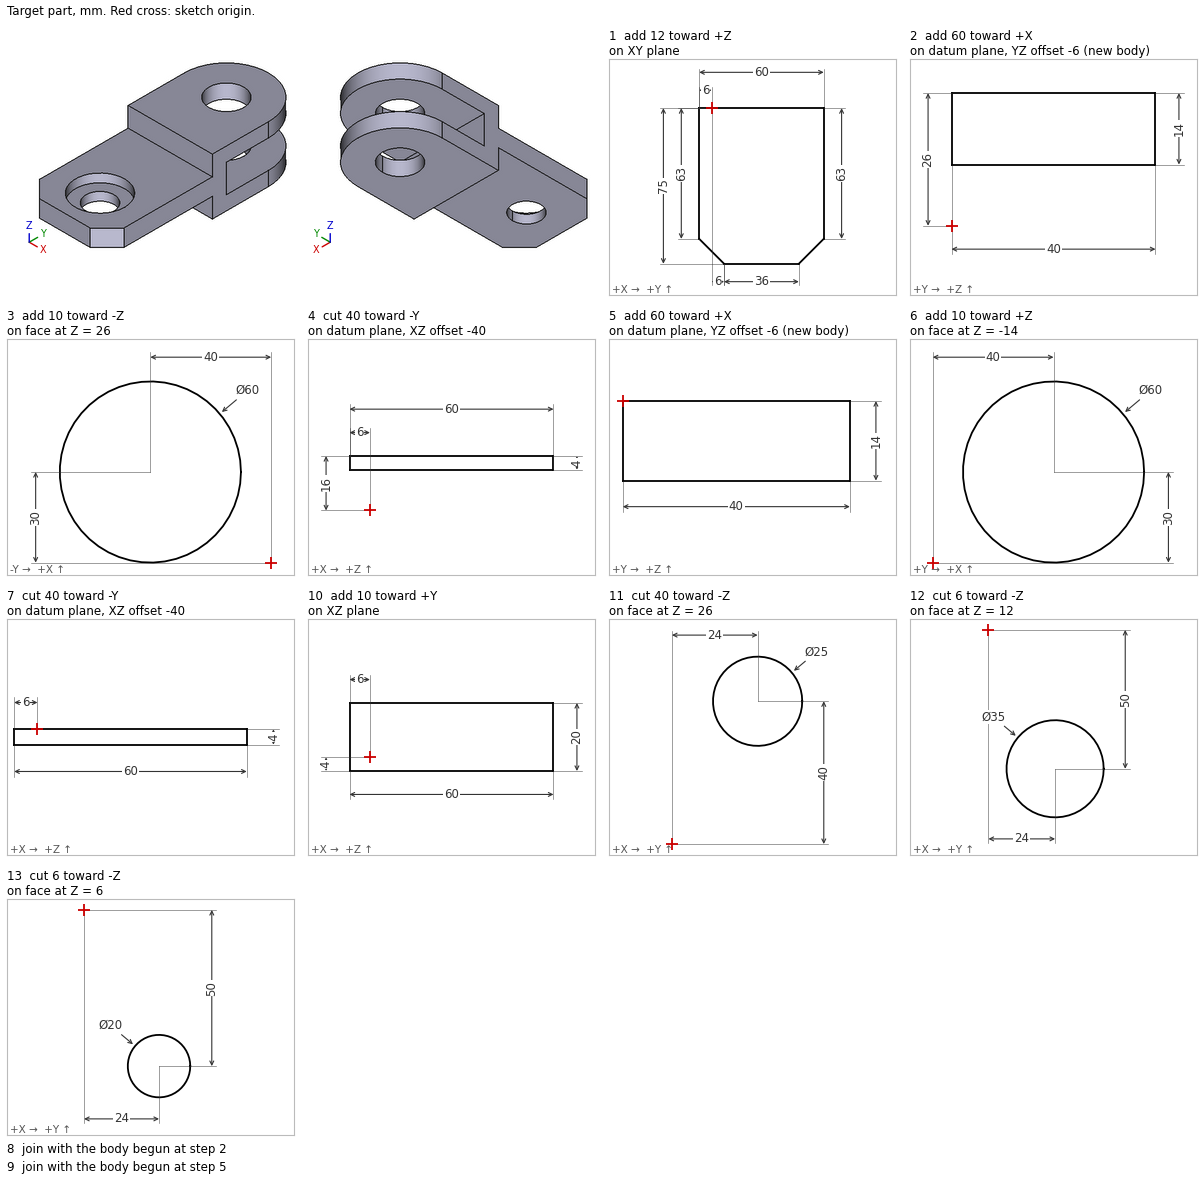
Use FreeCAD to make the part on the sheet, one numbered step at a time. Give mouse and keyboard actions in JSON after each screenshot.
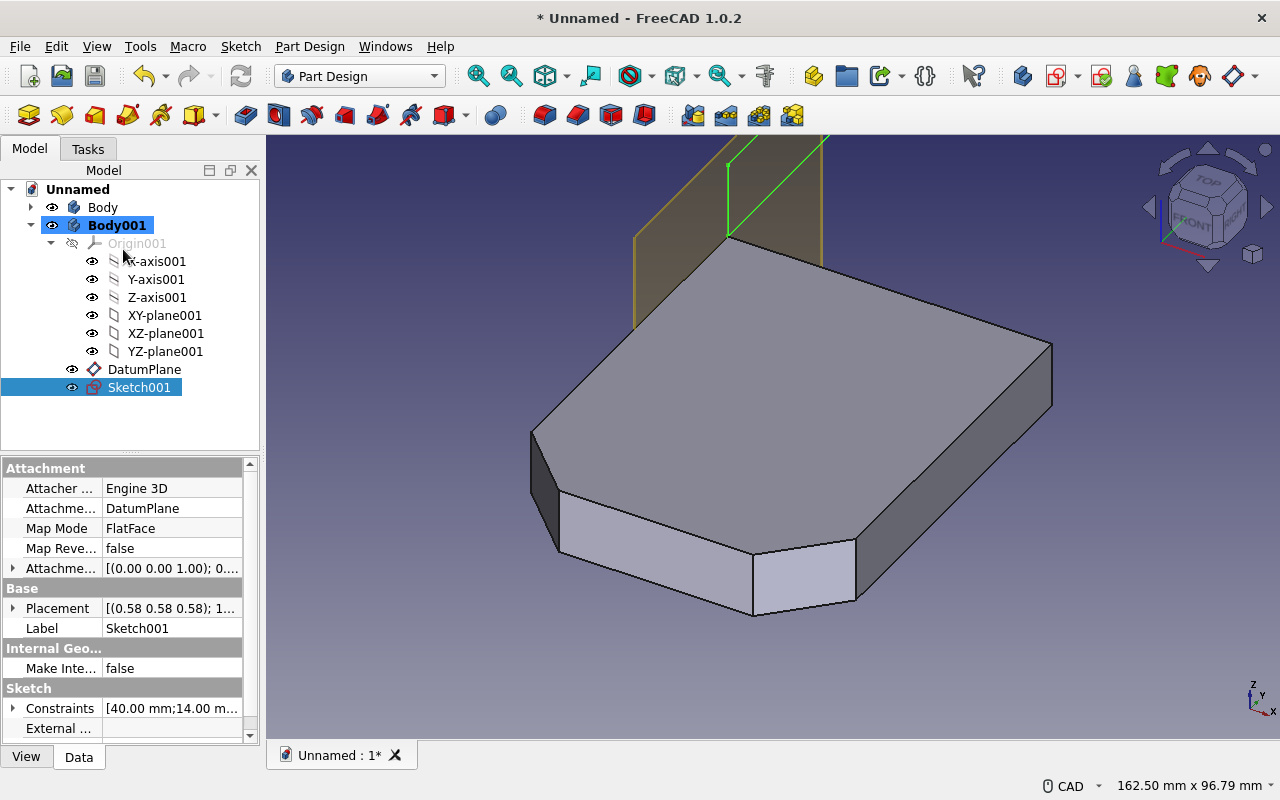
{"action": "left_click", "coordinate": [29, 116]}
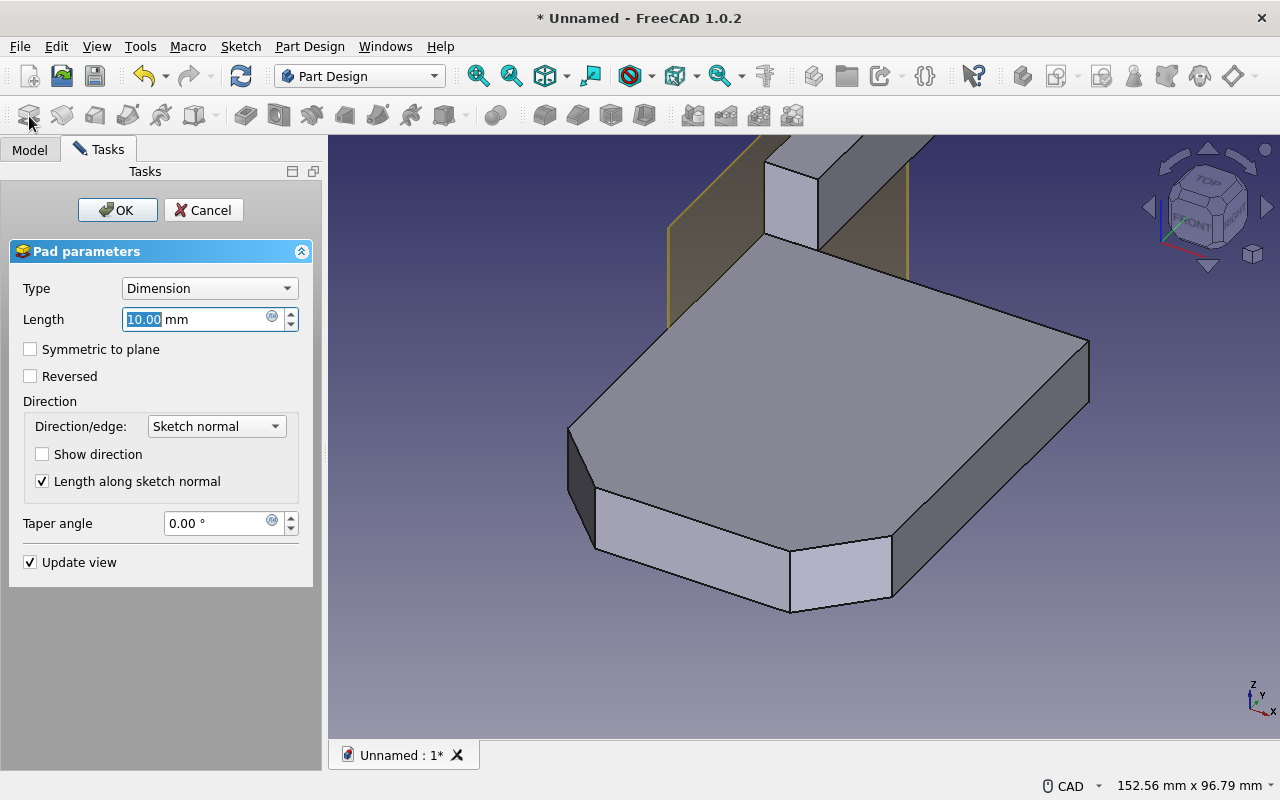
{"action": "type", "text": "60"}
{"action": "key", "text": "Tab"}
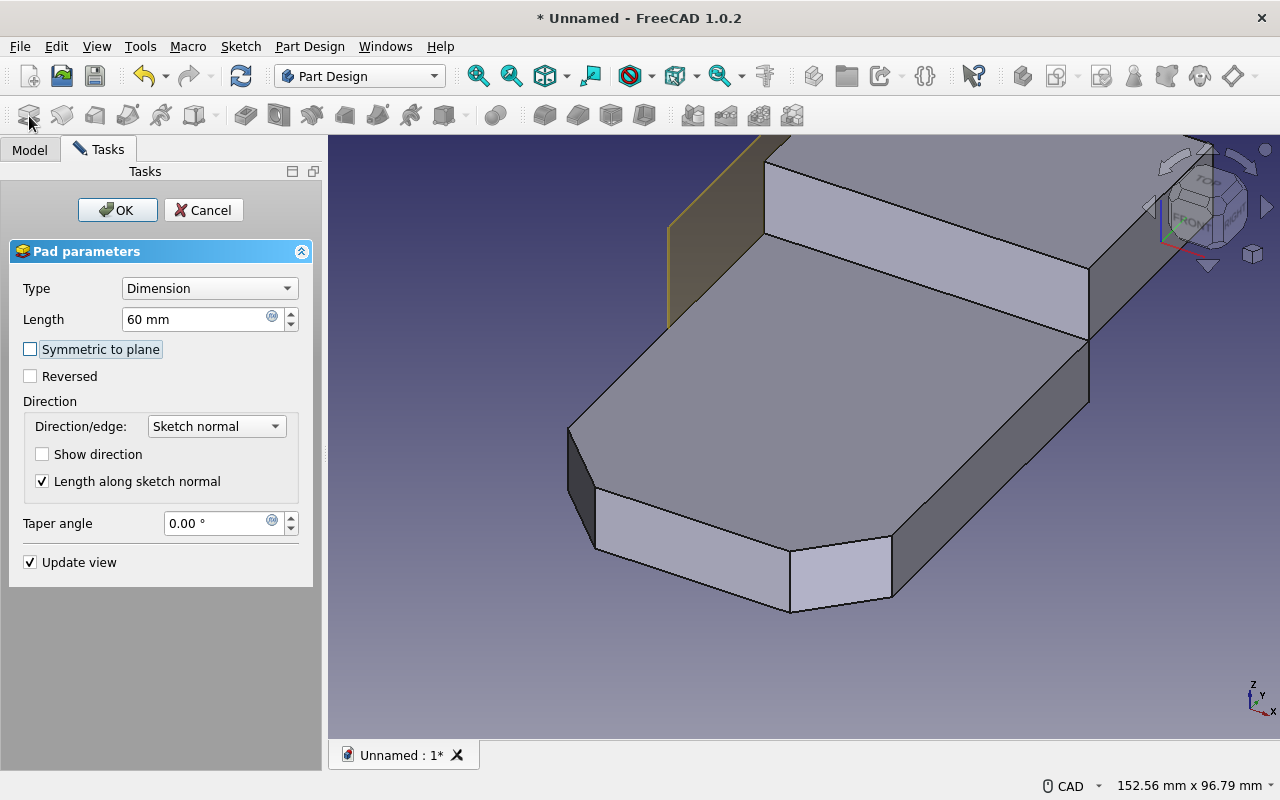
{"action": "left_click", "coordinate": [118, 210]}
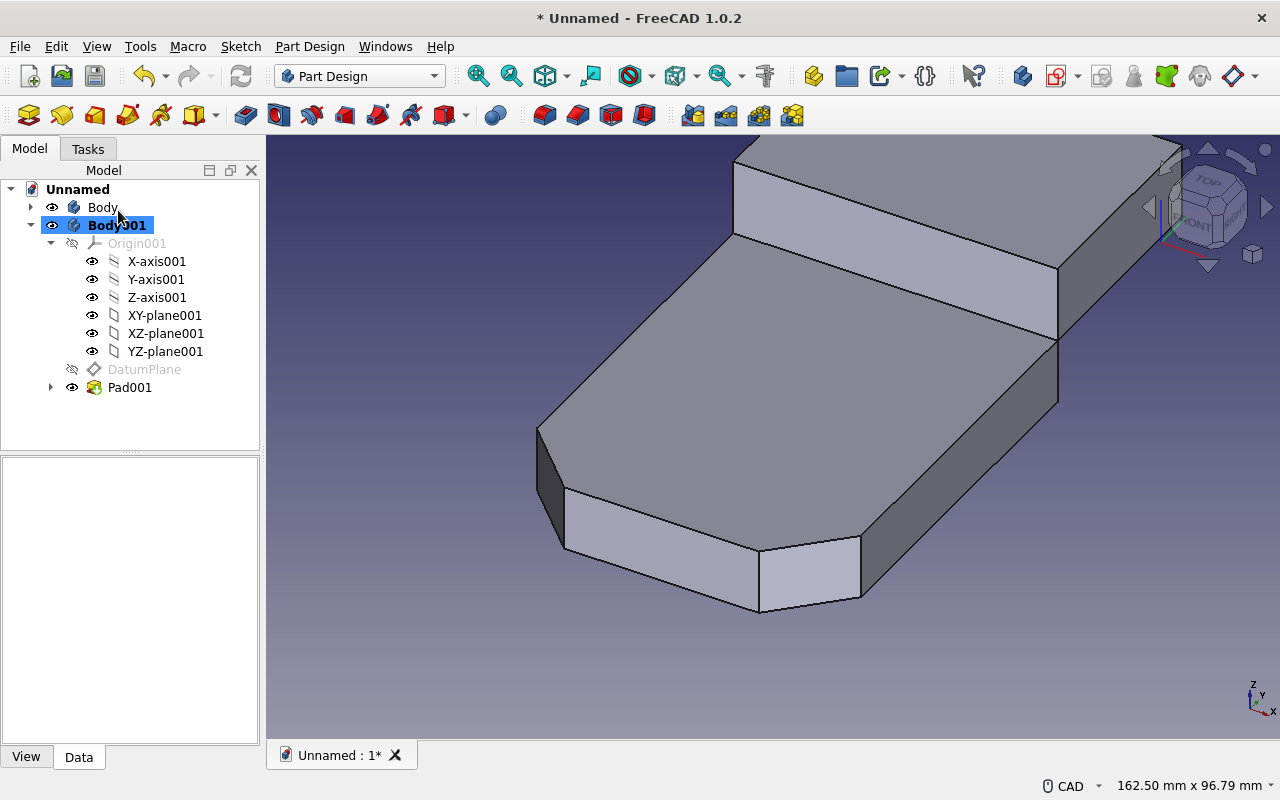
{"action": "left_click", "coordinate": [479, 76]}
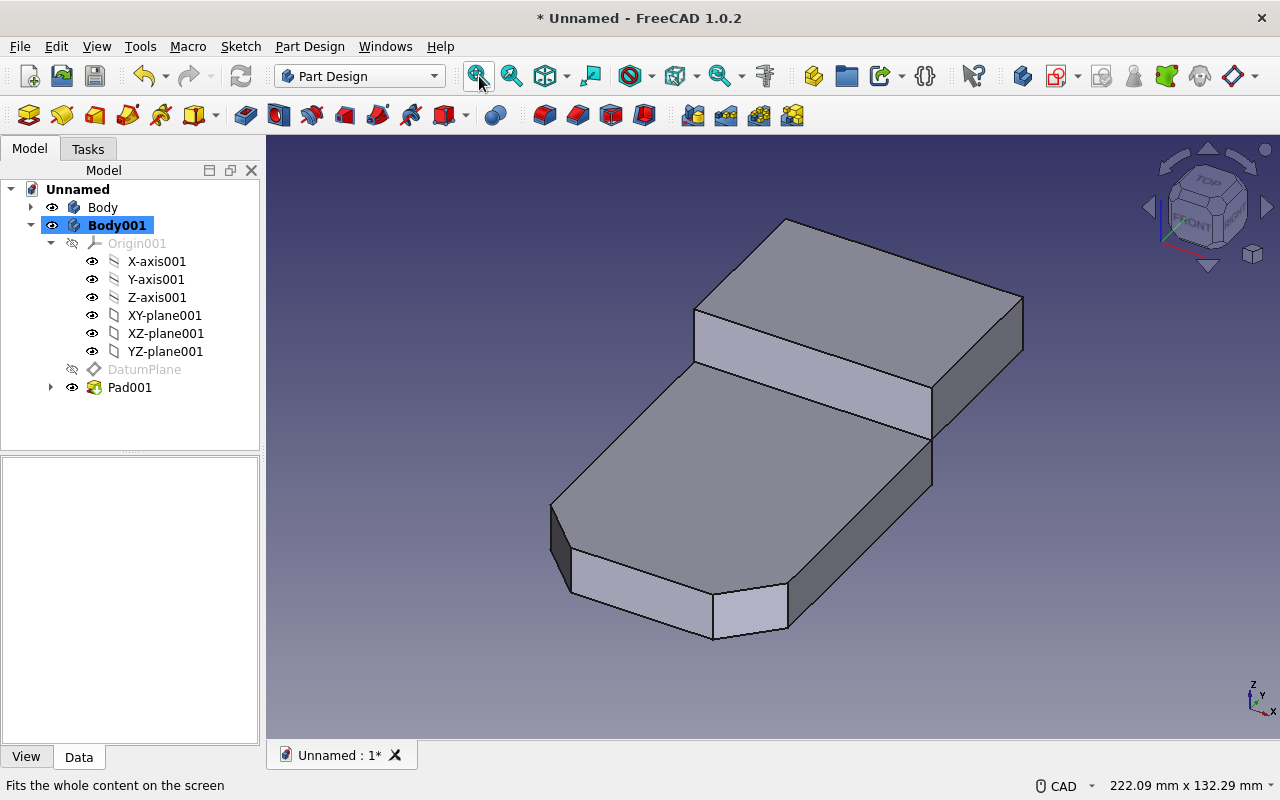
{"action": "left_click", "coordinate": [892, 314]}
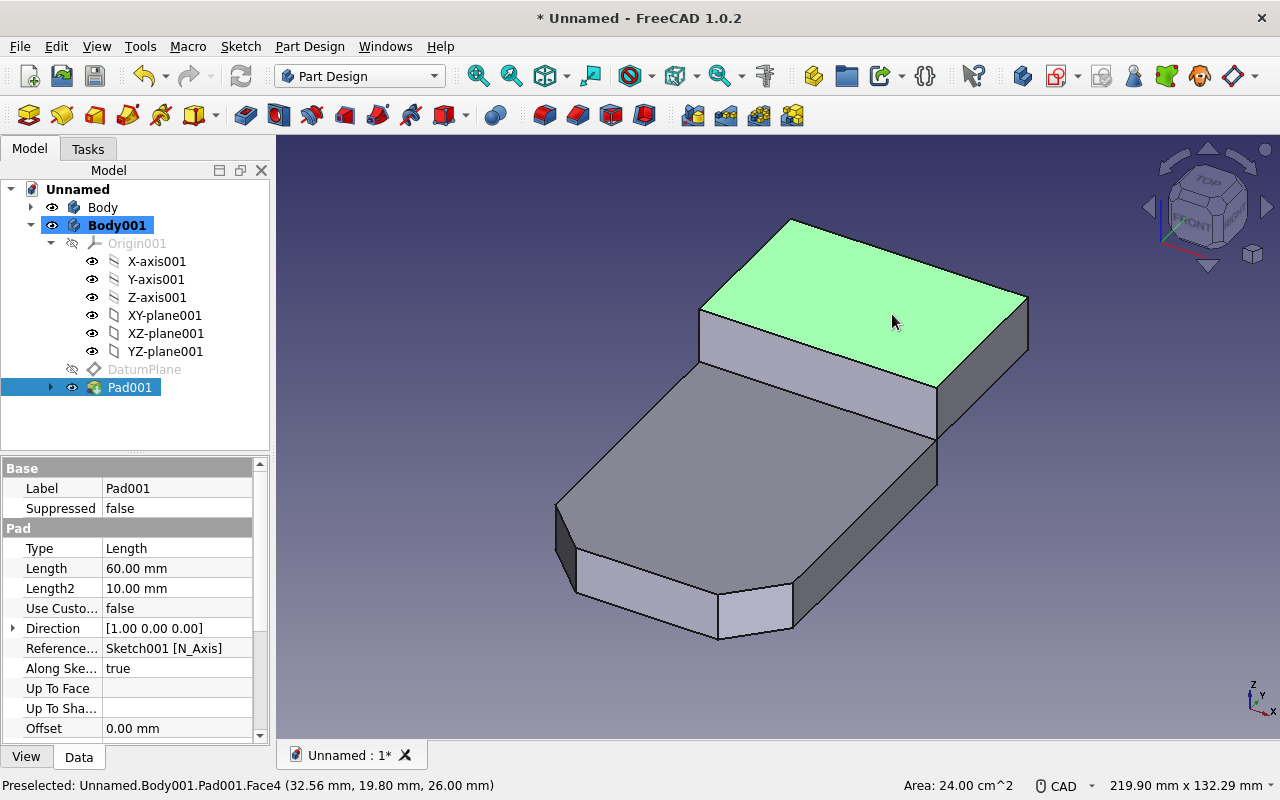
{"action": "left_click", "coordinate": [1056, 76]}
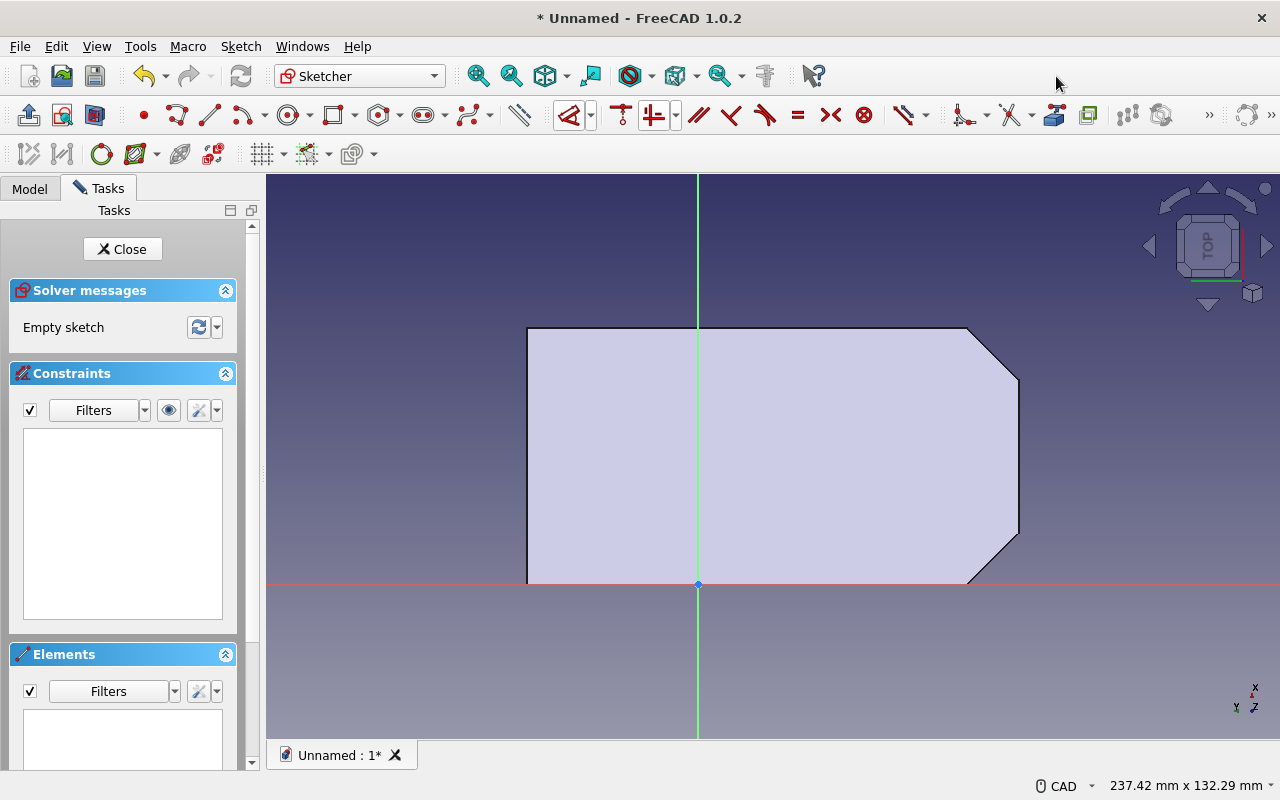
{"action": "scroll", "coordinate": [294, 457], "scroll_direction": "up", "scroll_amount": 2}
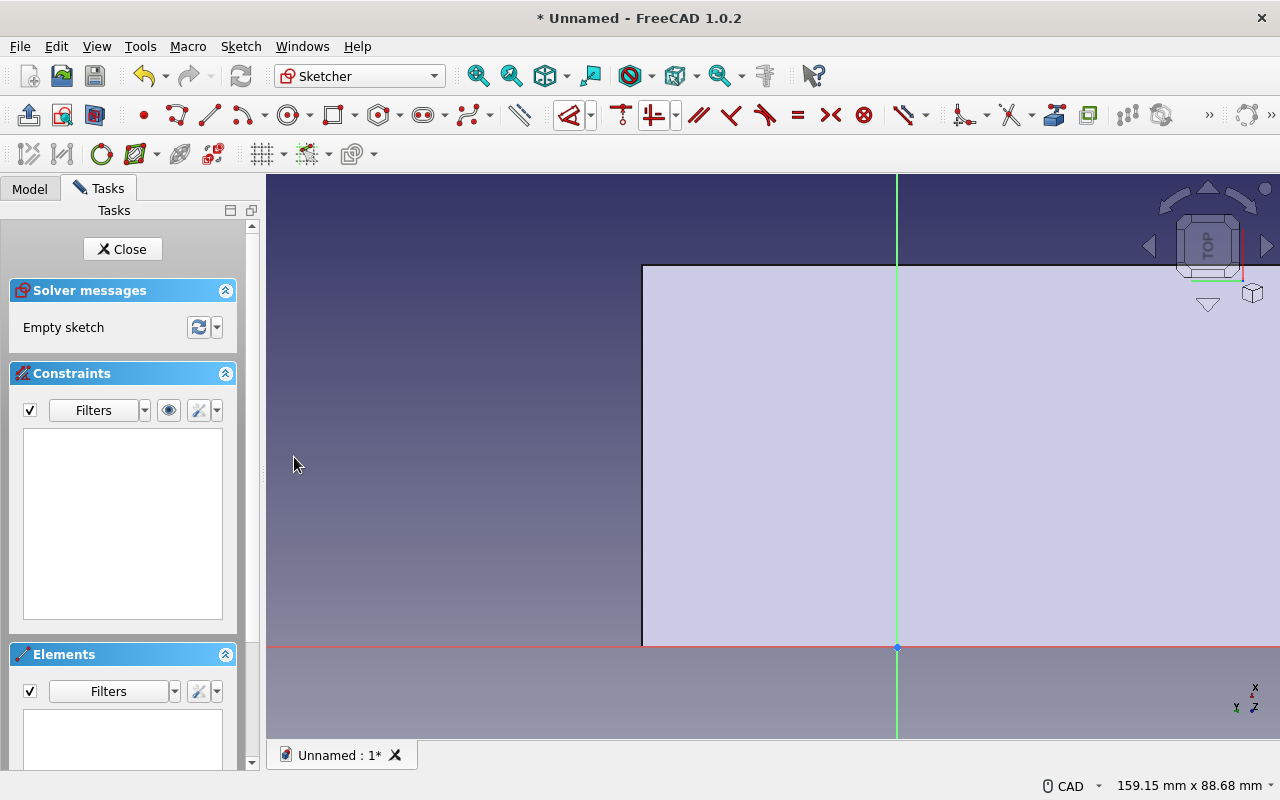
{"action": "left_click", "coordinate": [288, 116]}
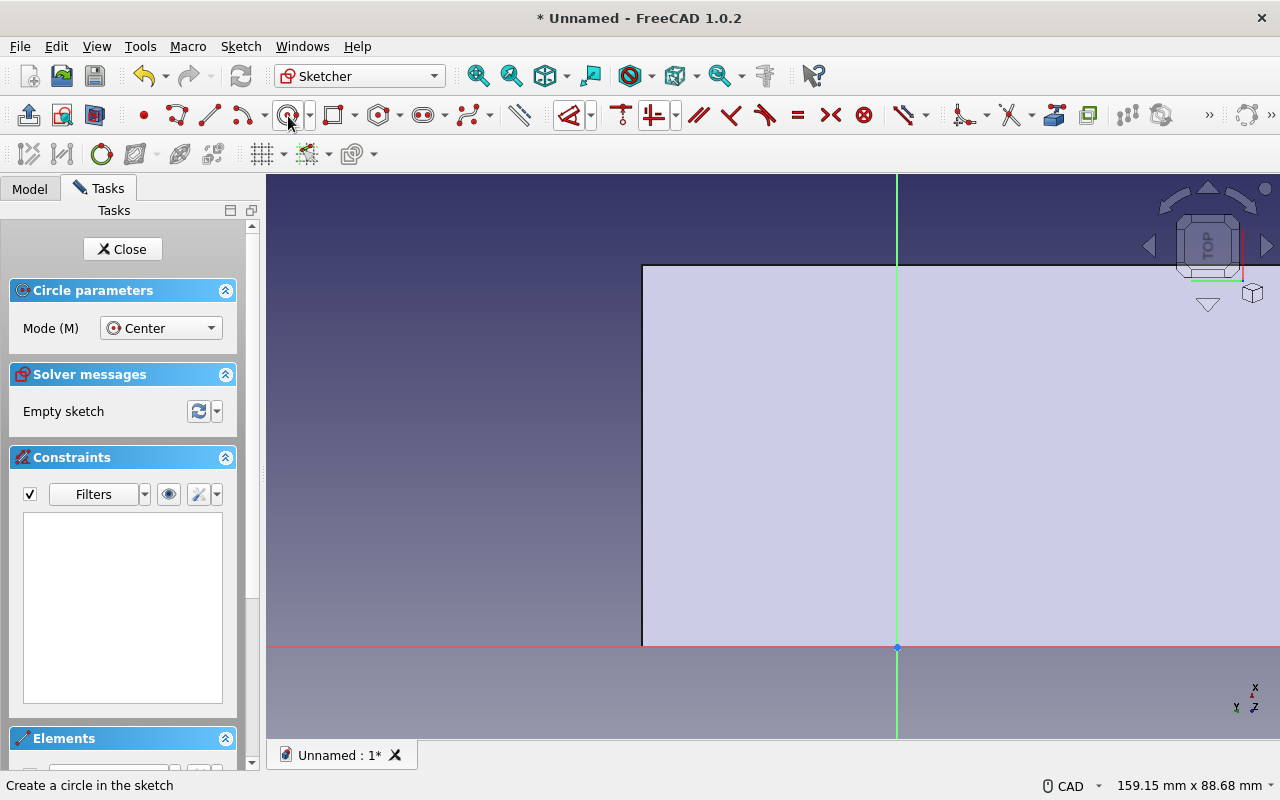
{"action": "left_click", "coordinate": [642, 456]}
{"action": "mouse_move", "coordinate": [777, 321]}